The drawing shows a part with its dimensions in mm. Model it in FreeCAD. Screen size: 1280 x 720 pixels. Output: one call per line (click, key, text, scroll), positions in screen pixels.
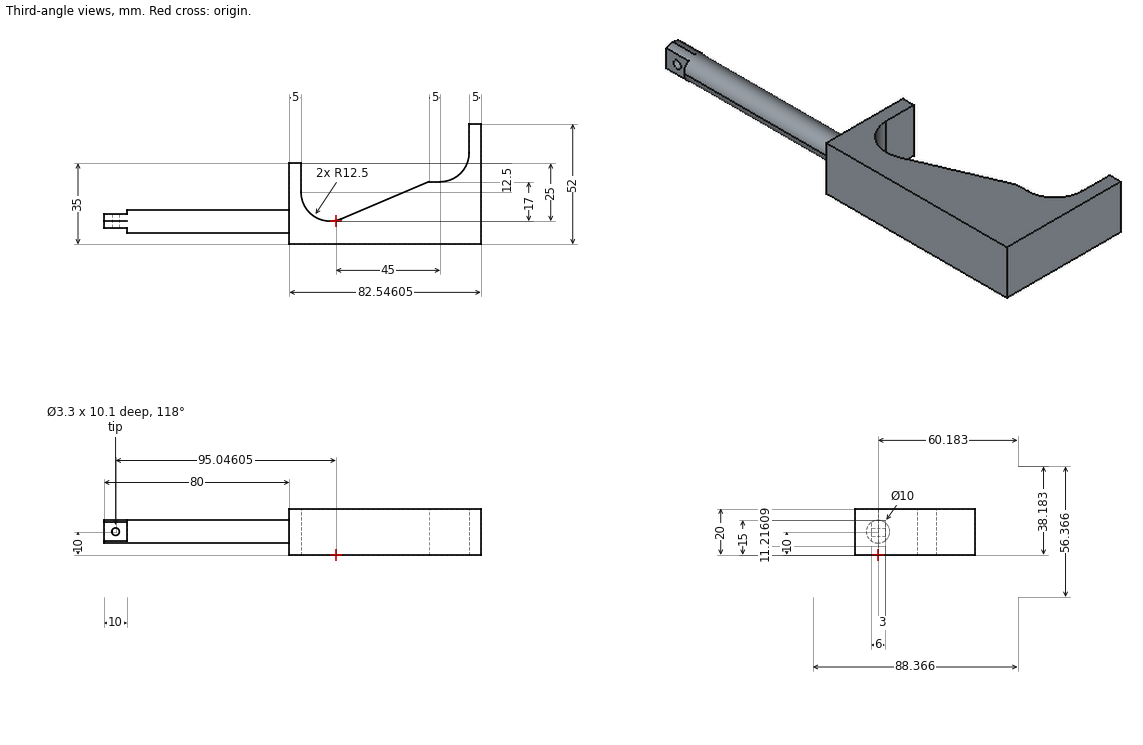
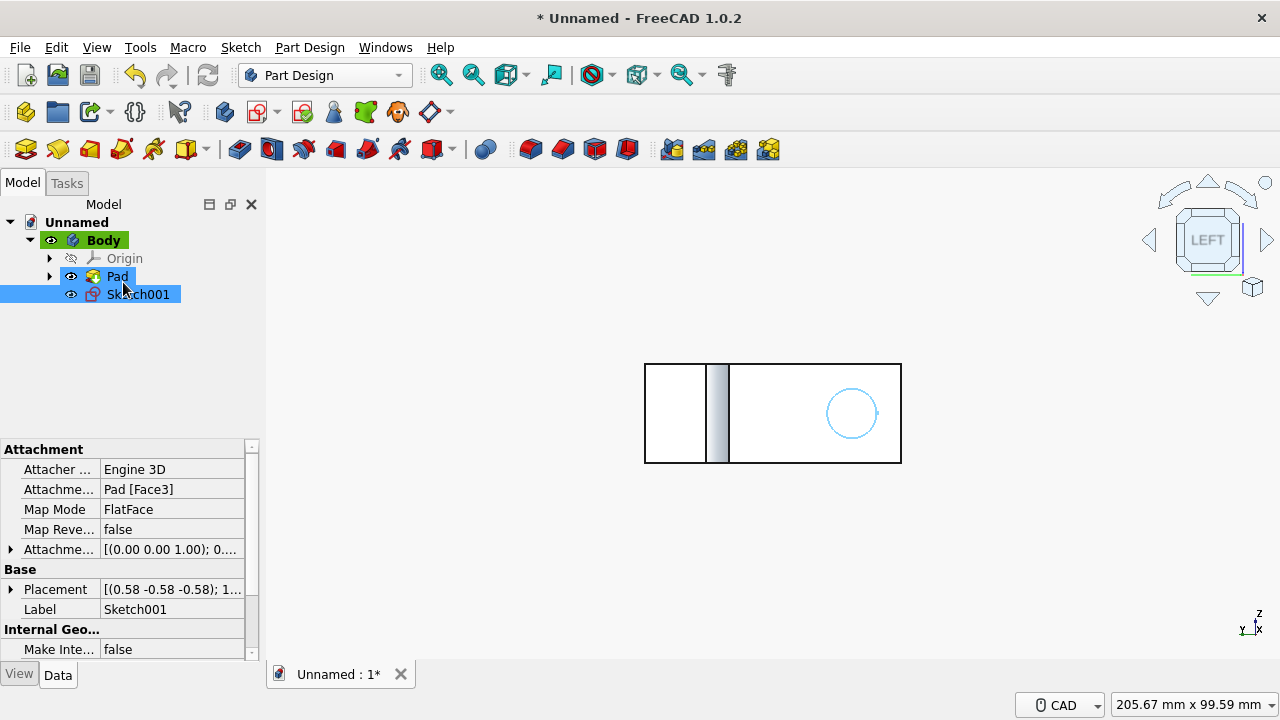
click(26, 150)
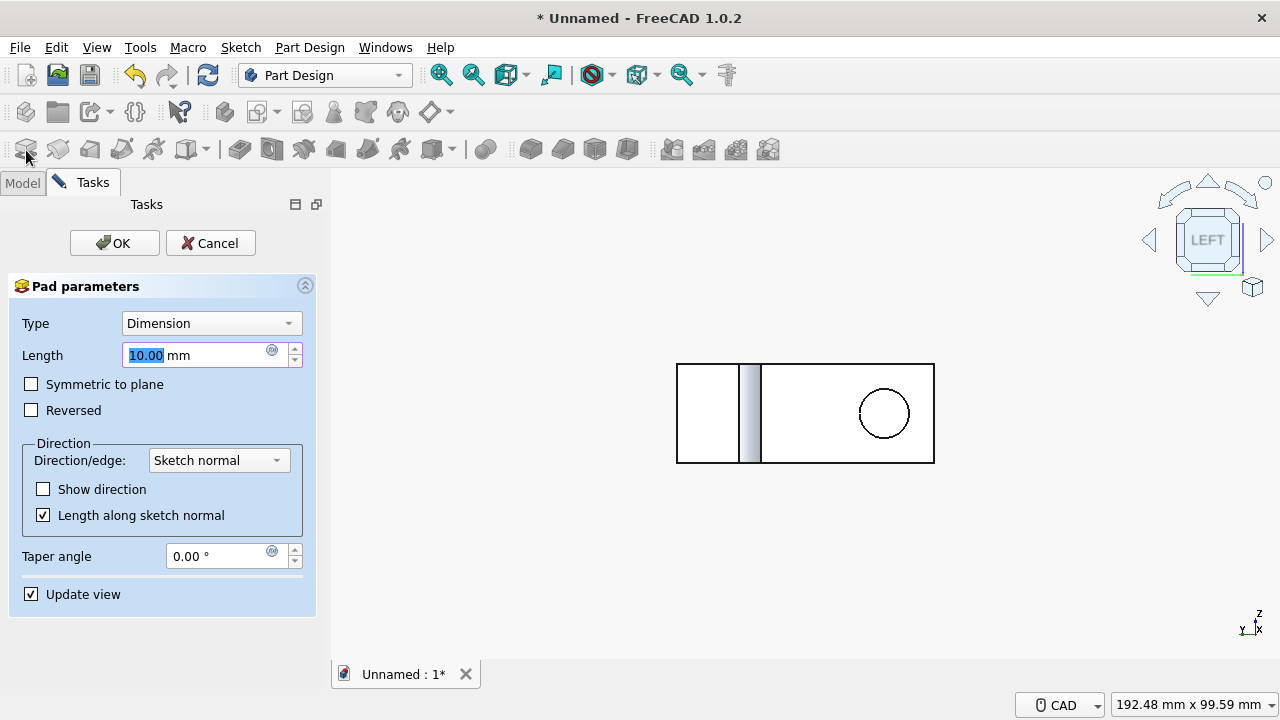
text(80)
key(Tab)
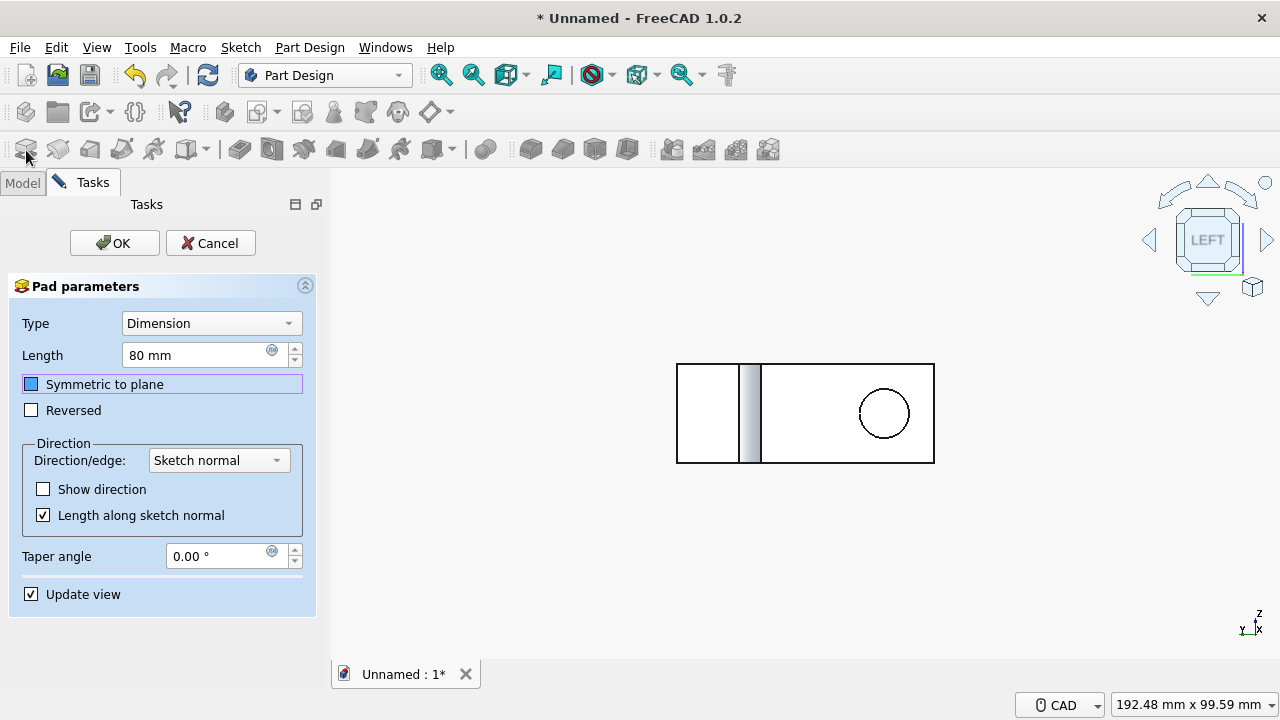
click(115, 243)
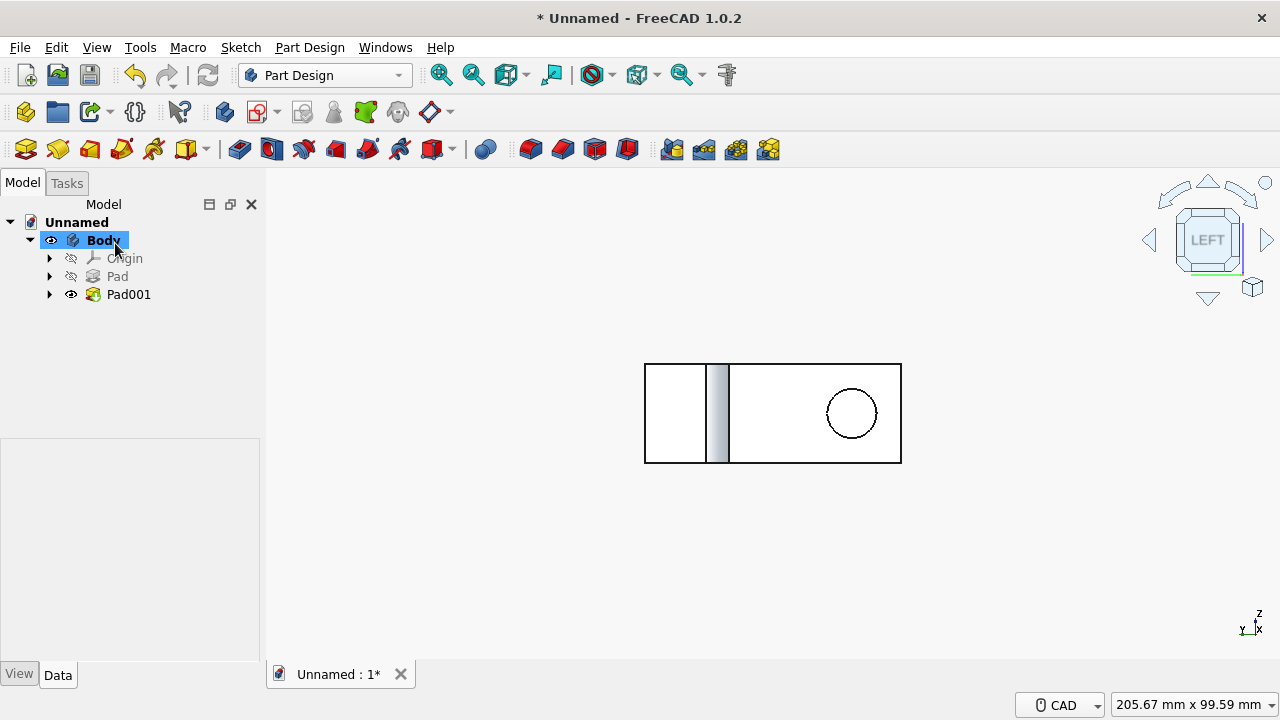
click(442, 76)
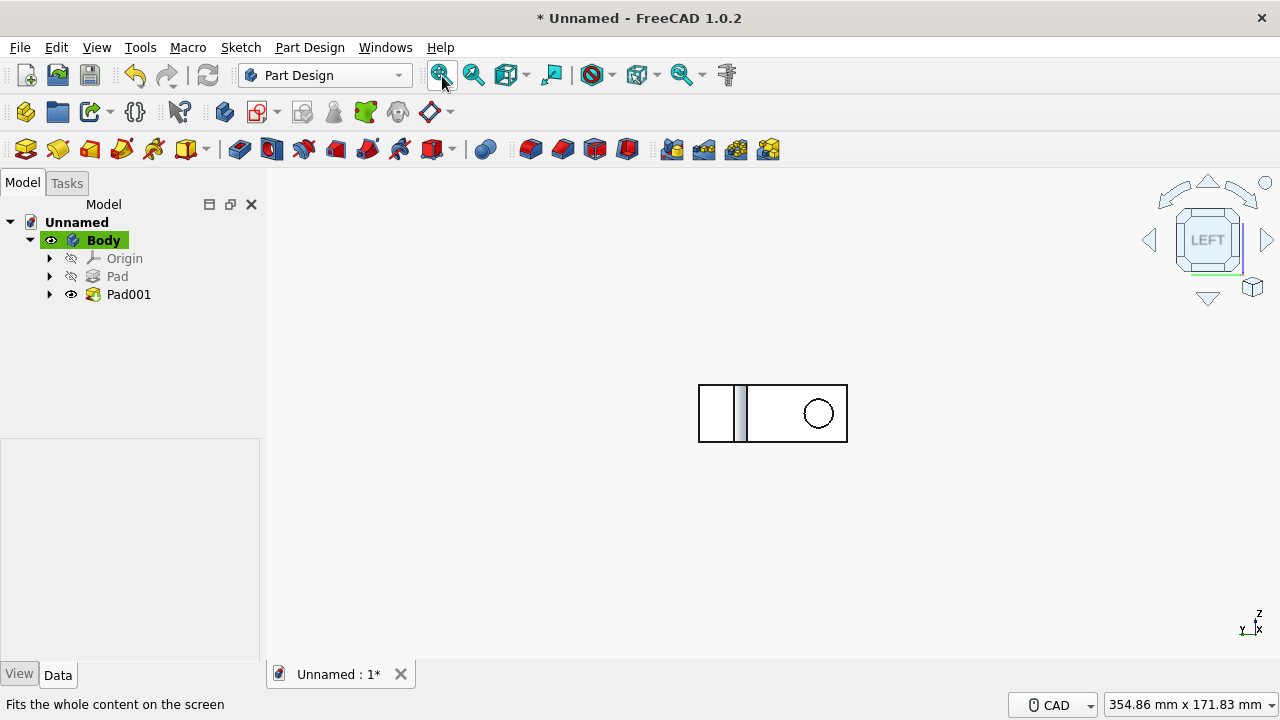
click(819, 412)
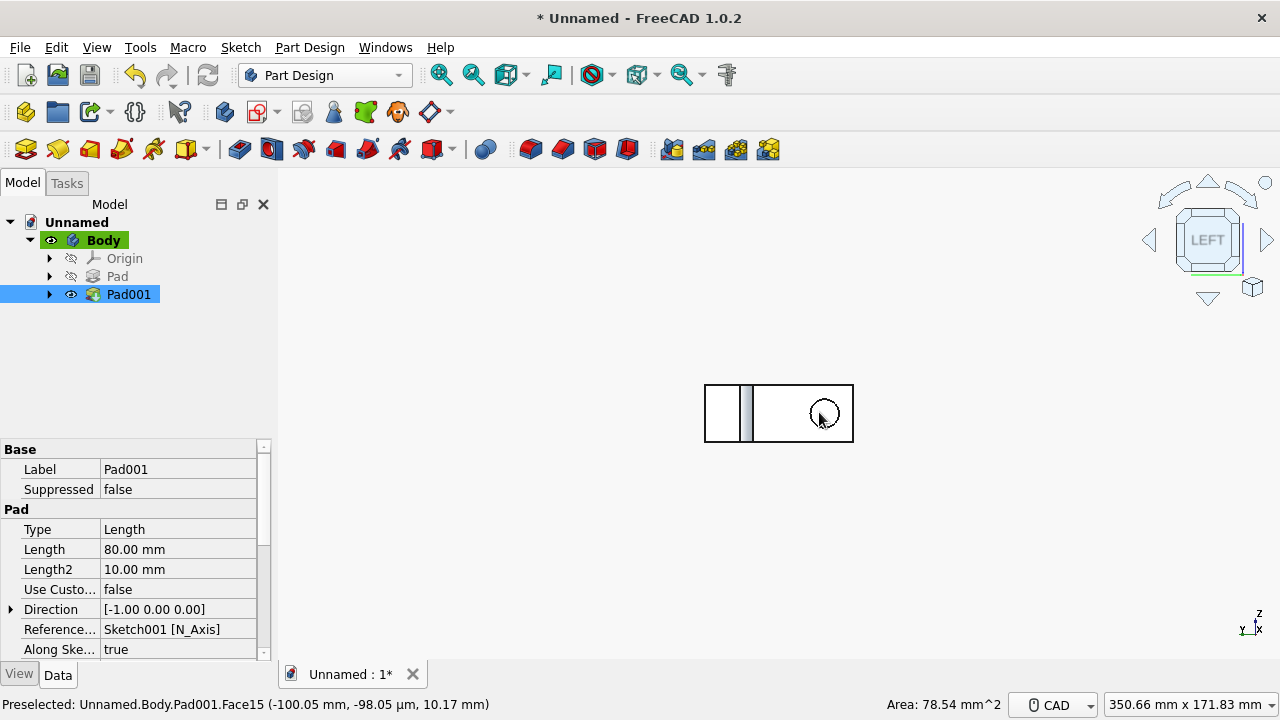
click(258, 112)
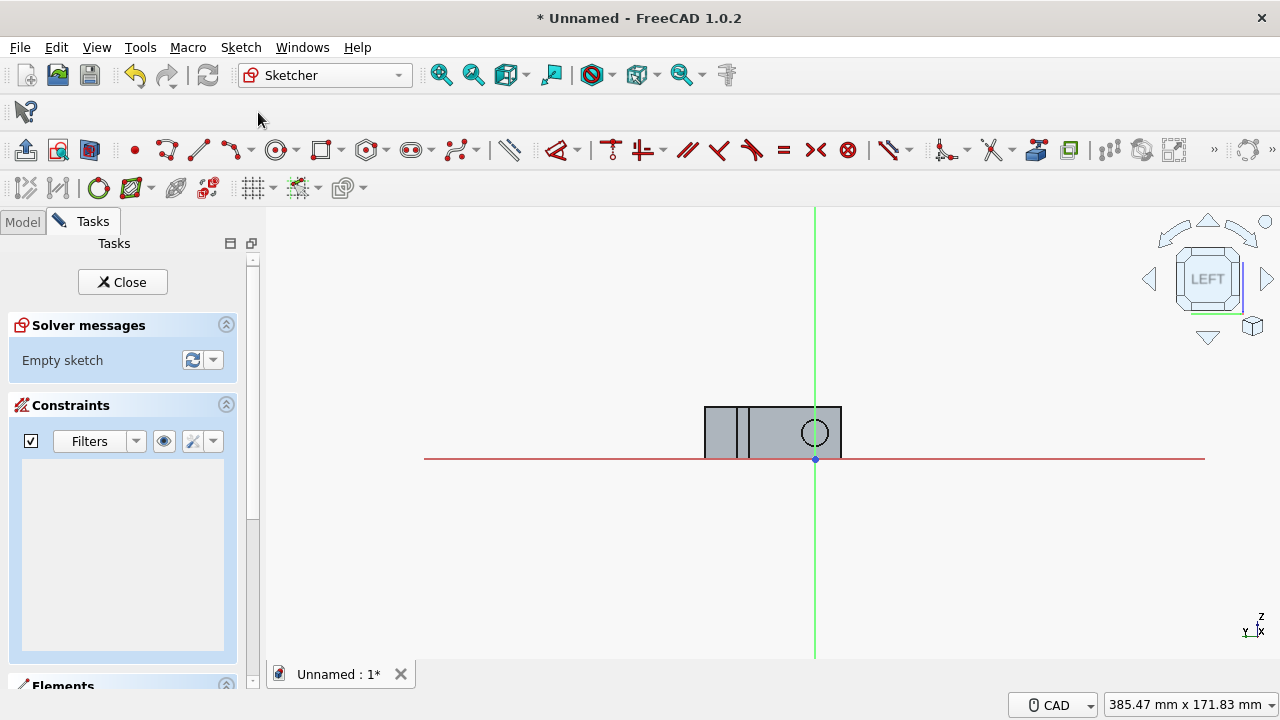
scroll(856, 433, up, 3)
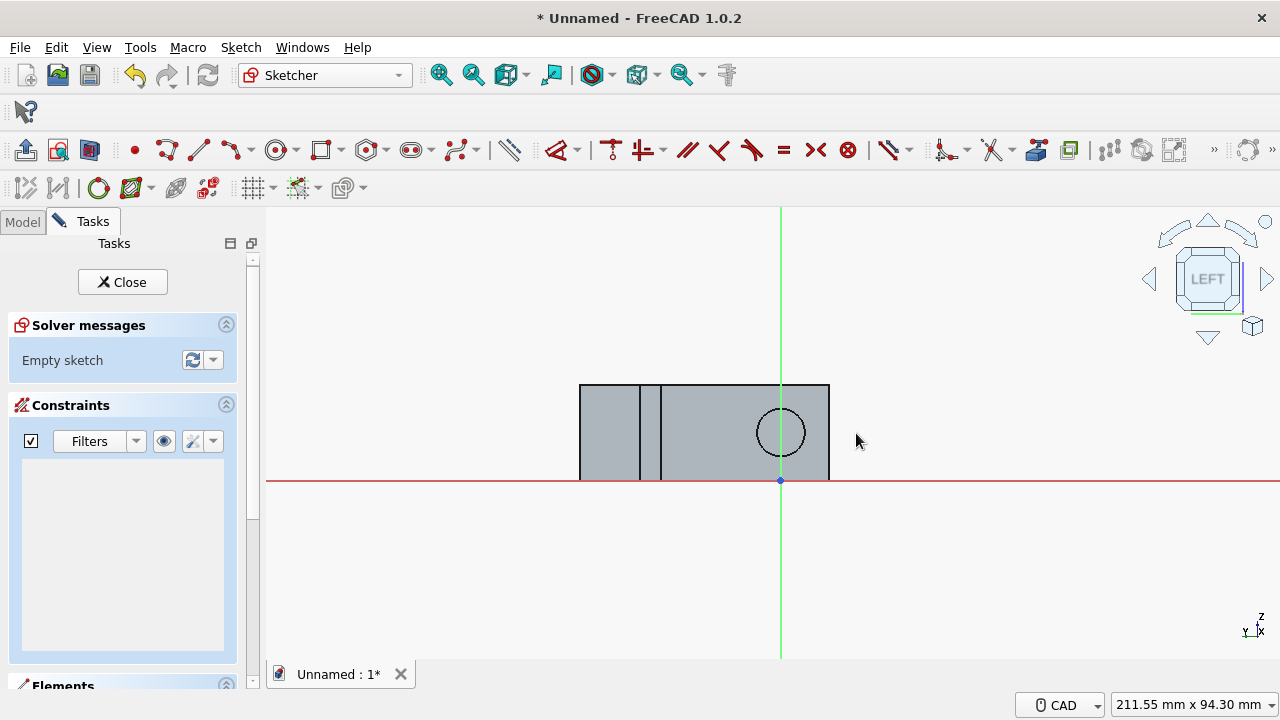
click(322, 150)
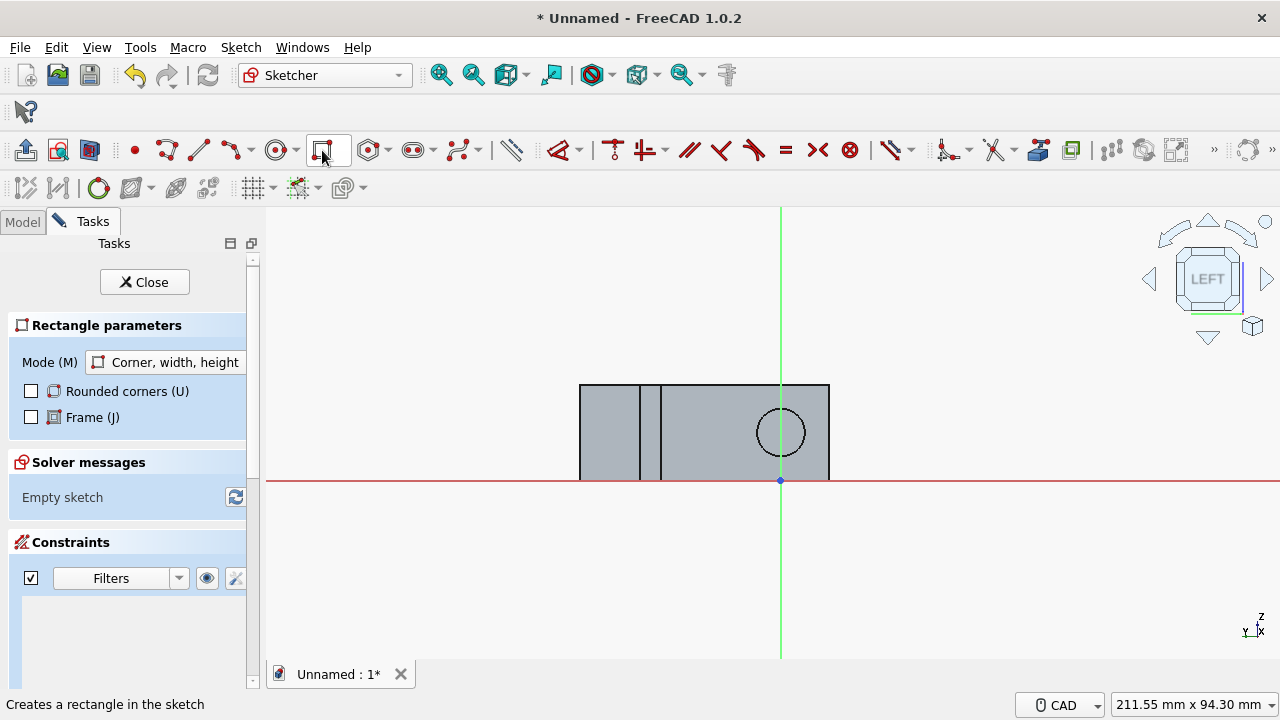
click(493, 298)
click(916, 568)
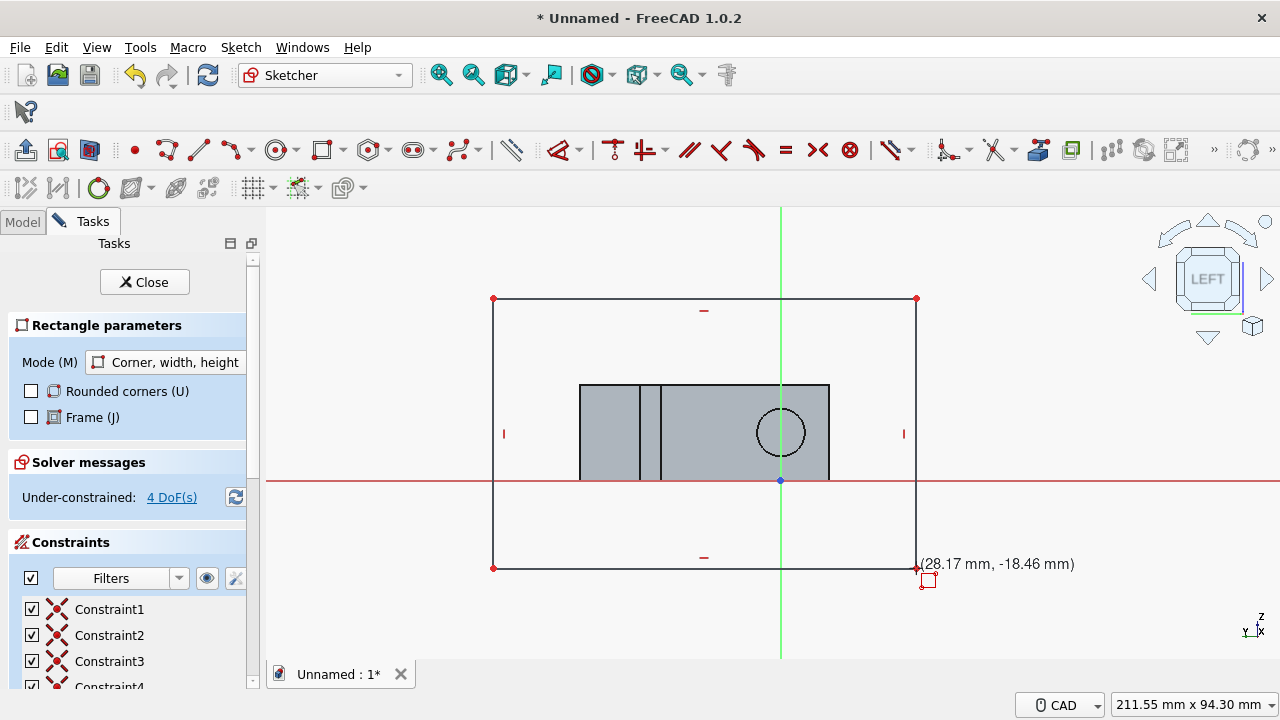
click(767, 409)
click(795, 462)
key(Escape)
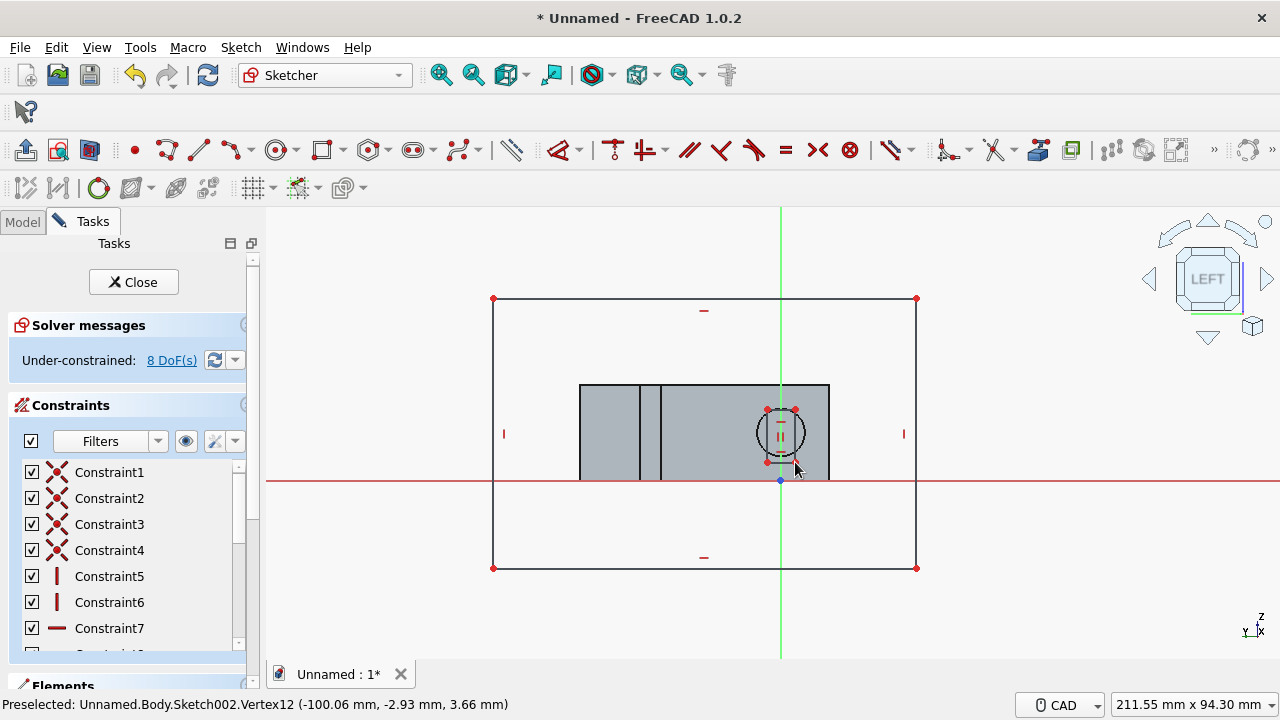
click(558, 150)